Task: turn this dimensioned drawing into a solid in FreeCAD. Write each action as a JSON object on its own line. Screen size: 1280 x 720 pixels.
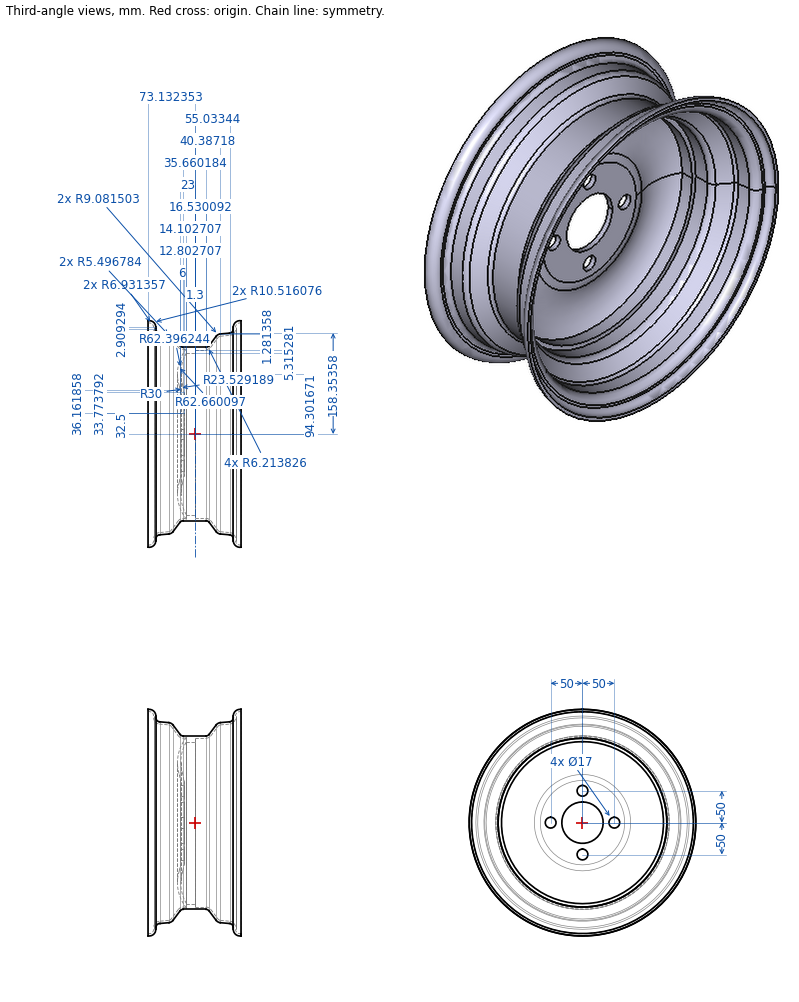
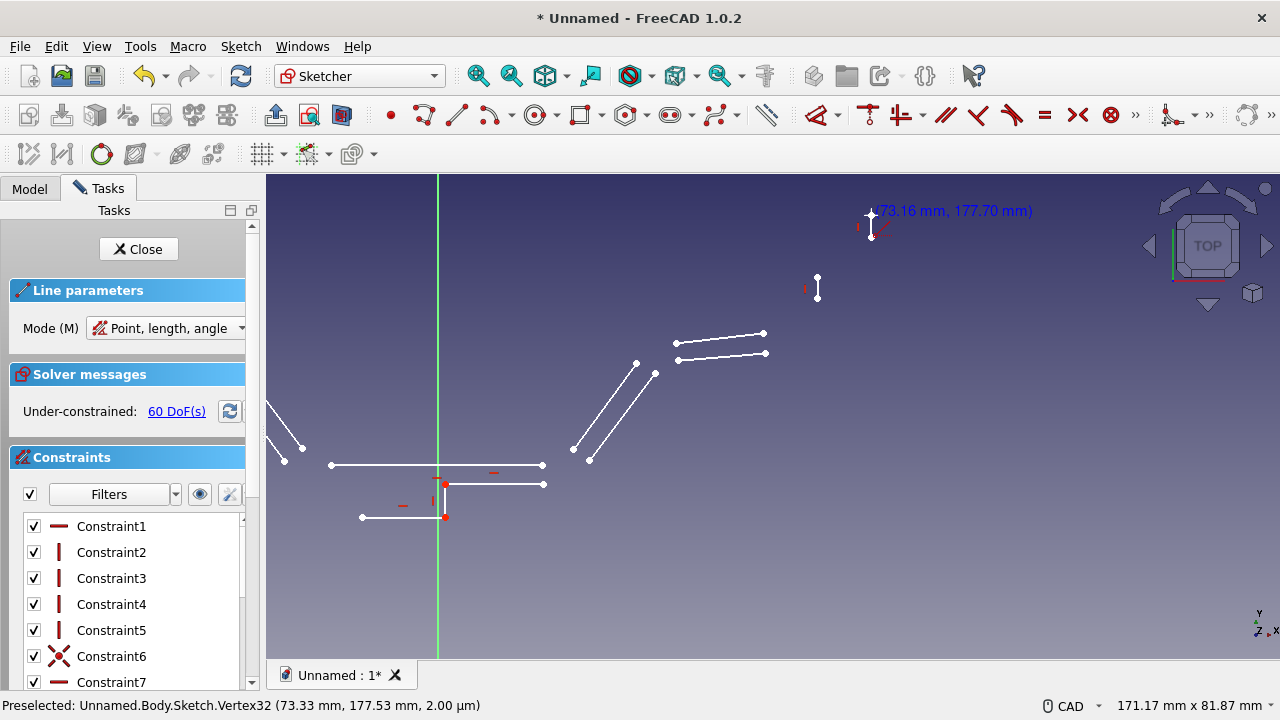
{"action": "left_click", "coordinate": [797, 277]}
{"action": "left_click", "coordinate": [797, 294]}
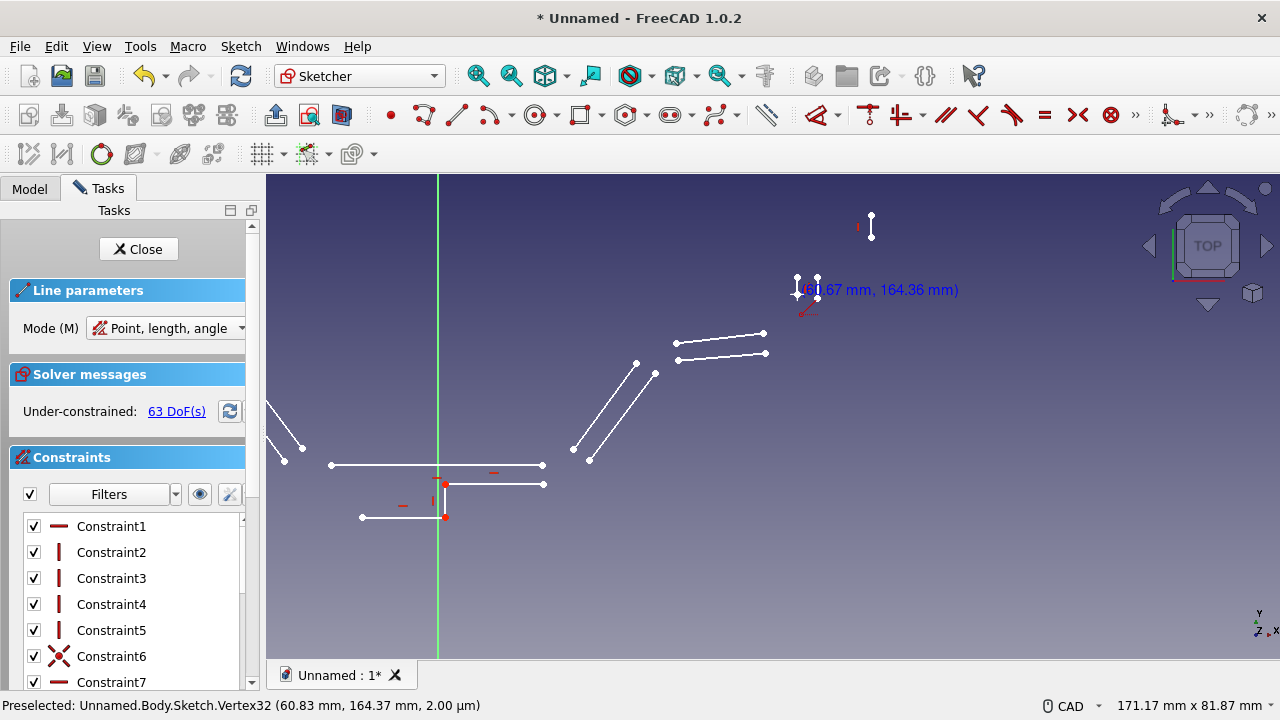
{"action": "key", "text": "g 3 a"}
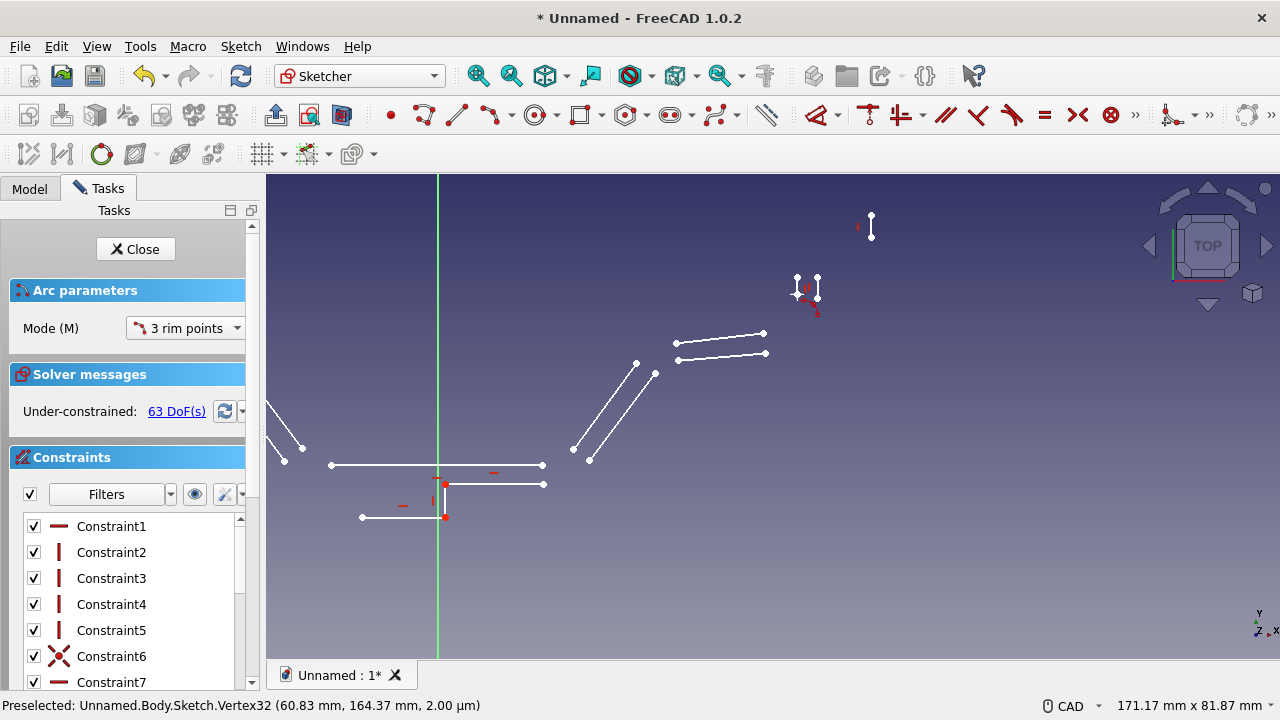
{"action": "left_click", "coordinate": [677, 343]}
{"action": "left_click", "coordinate": [637, 363]}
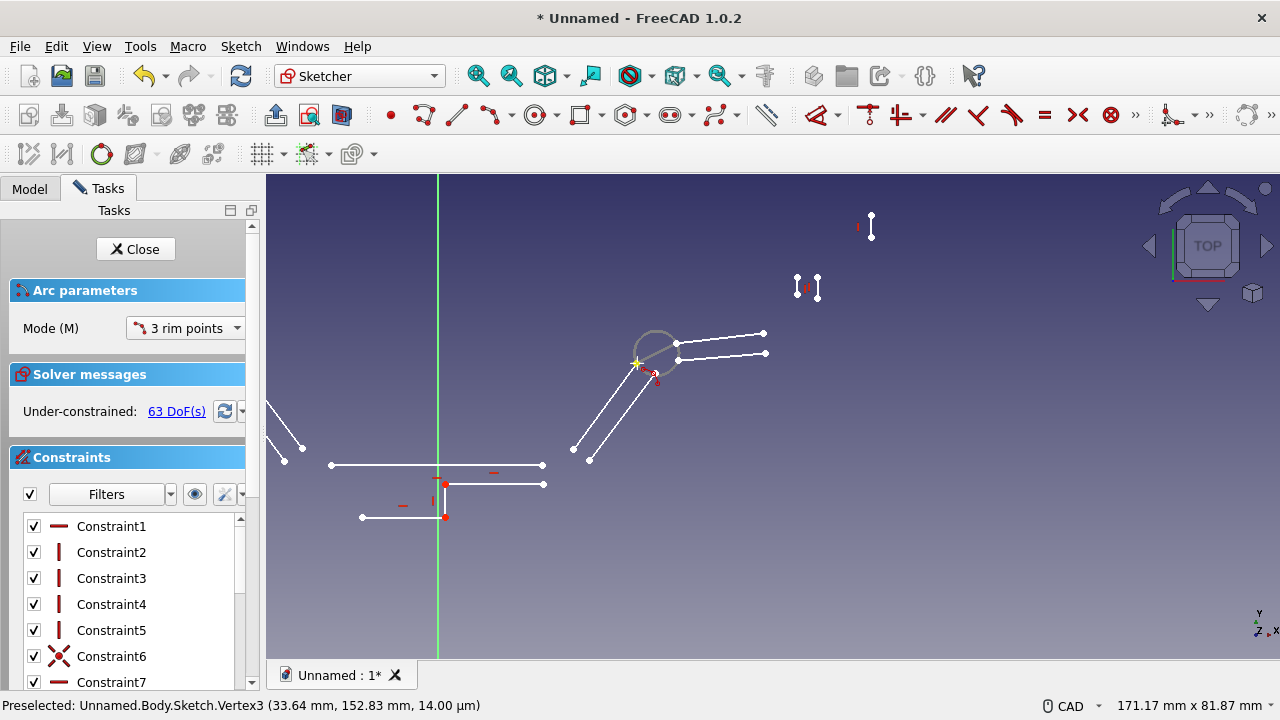
{"action": "scroll", "coordinate": [655, 345], "scroll_direction": "up", "scroll_amount": 7}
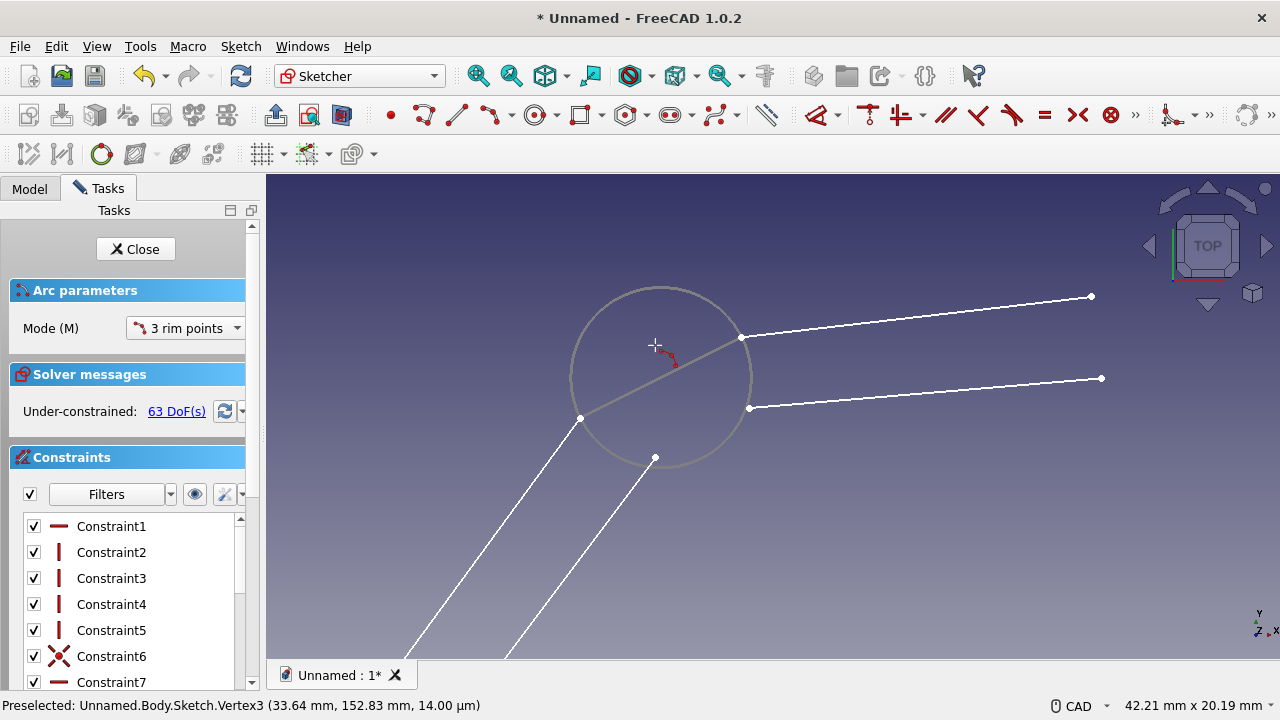
{"action": "left_click", "coordinate": [655, 343]}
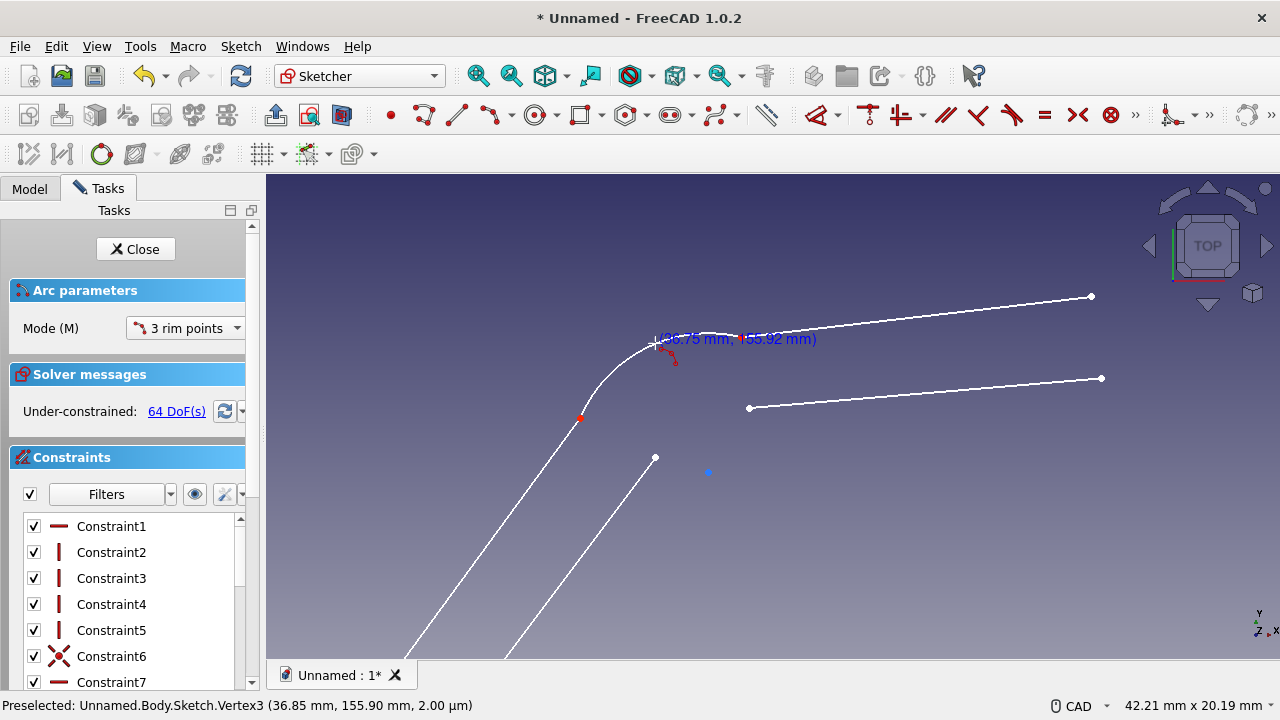
{"action": "scroll", "coordinate": [779, 293], "scroll_direction": "down", "scroll_amount": 13}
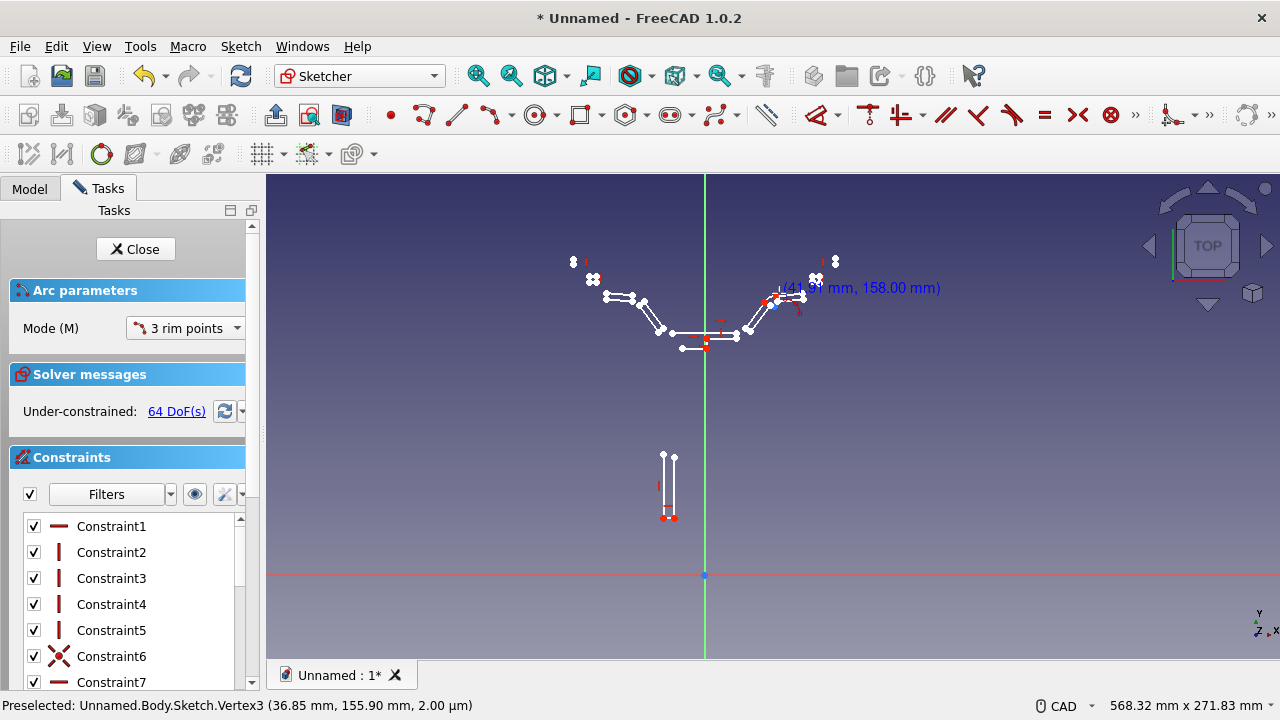
{"action": "scroll", "coordinate": [745, 328], "scroll_direction": "up", "scroll_amount": 5}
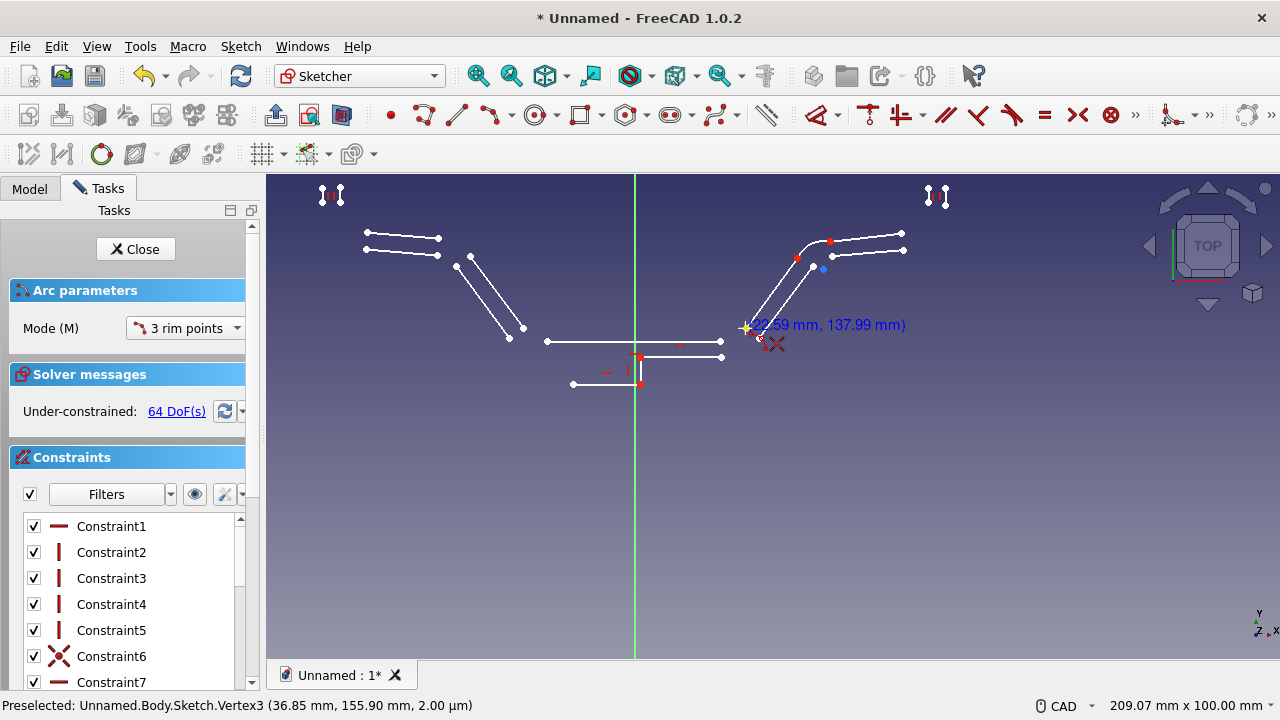
{"action": "left_click", "coordinate": [746, 329]}
{"action": "left_click", "coordinate": [721, 342]}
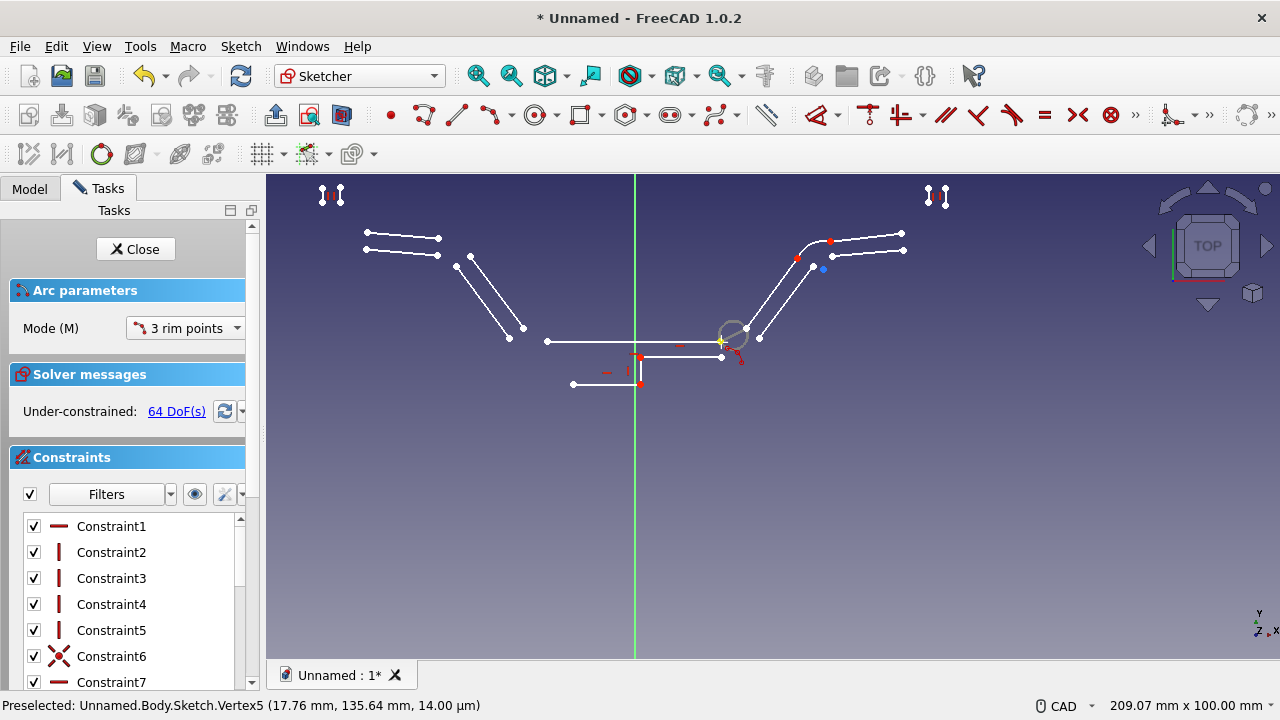
{"action": "scroll", "coordinate": [735, 336], "scroll_direction": "up", "scroll_amount": 9}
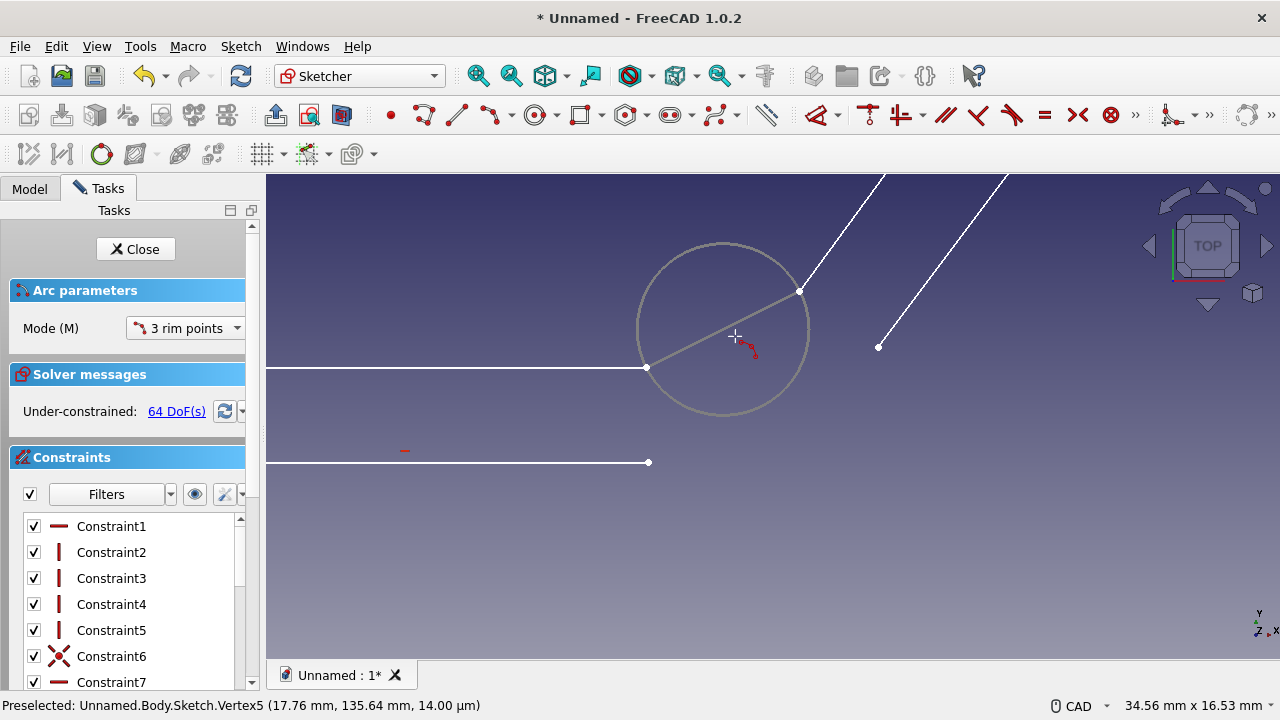
{"action": "left_click", "coordinate": [730, 335]}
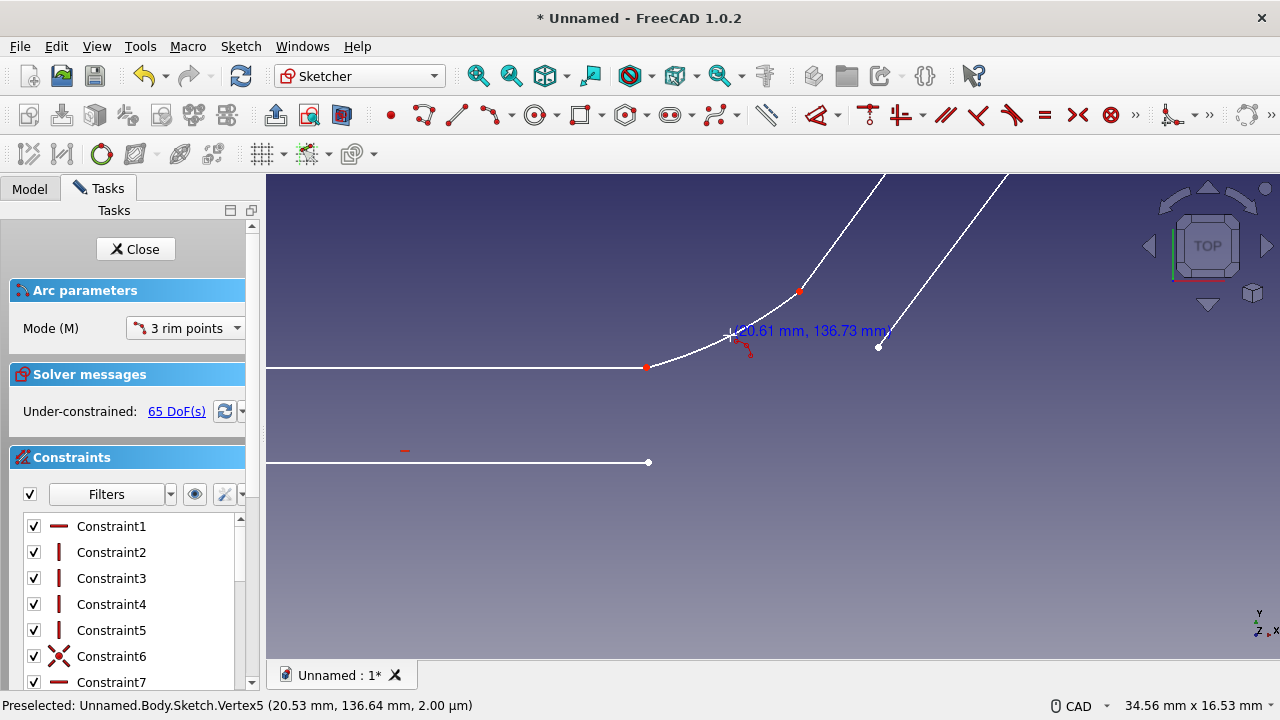
{"action": "scroll", "coordinate": [742, 331], "scroll_direction": "down", "scroll_amount": 14}